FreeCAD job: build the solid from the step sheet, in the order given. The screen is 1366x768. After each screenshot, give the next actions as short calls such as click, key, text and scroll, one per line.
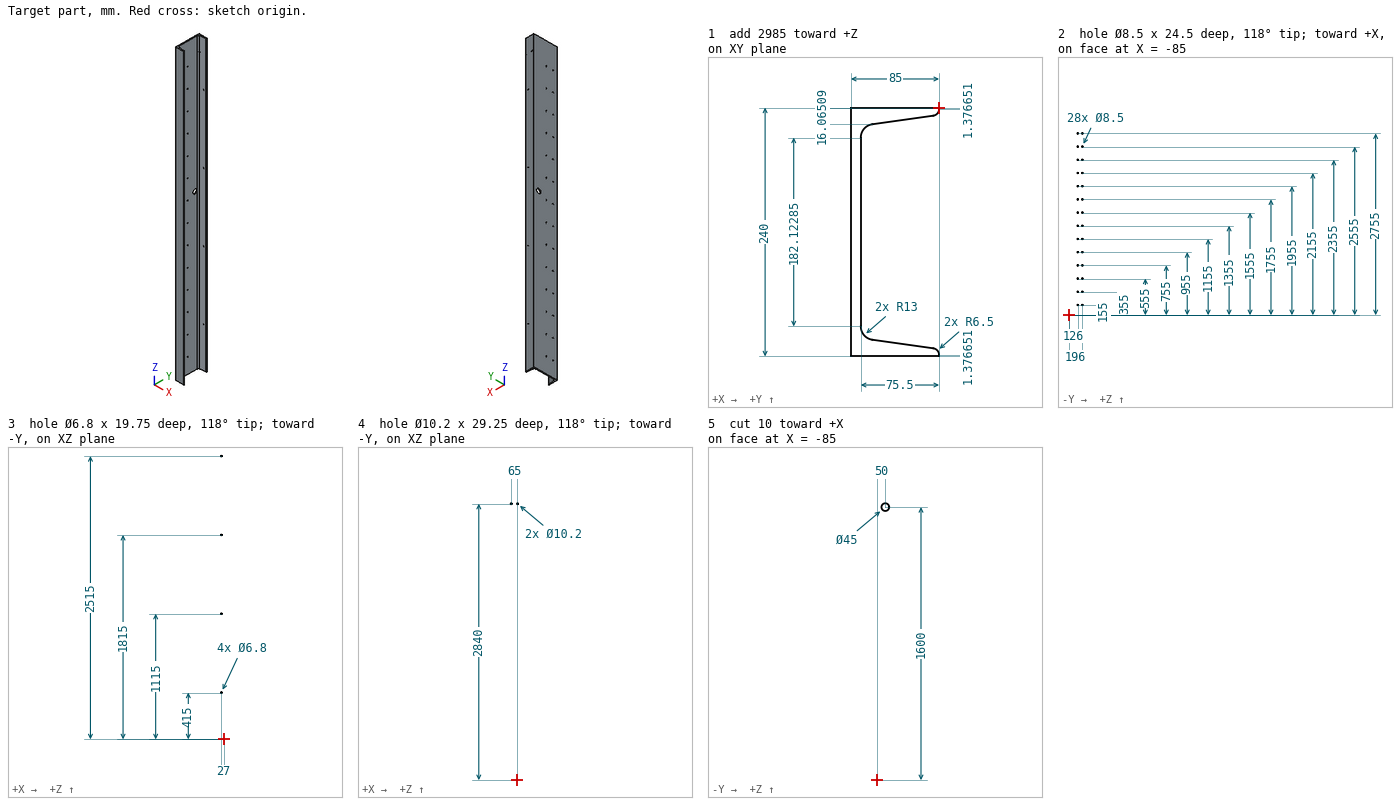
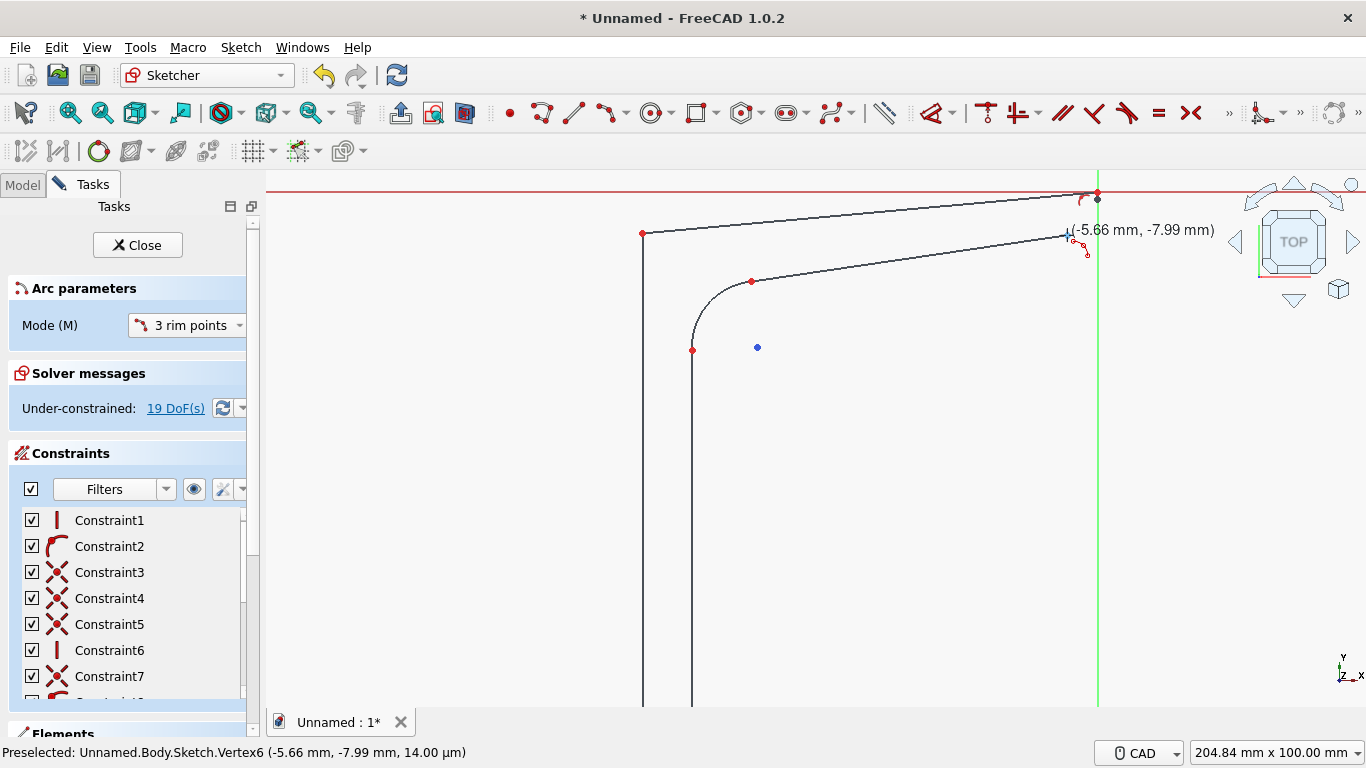
scroll(1098, 200, up, 8)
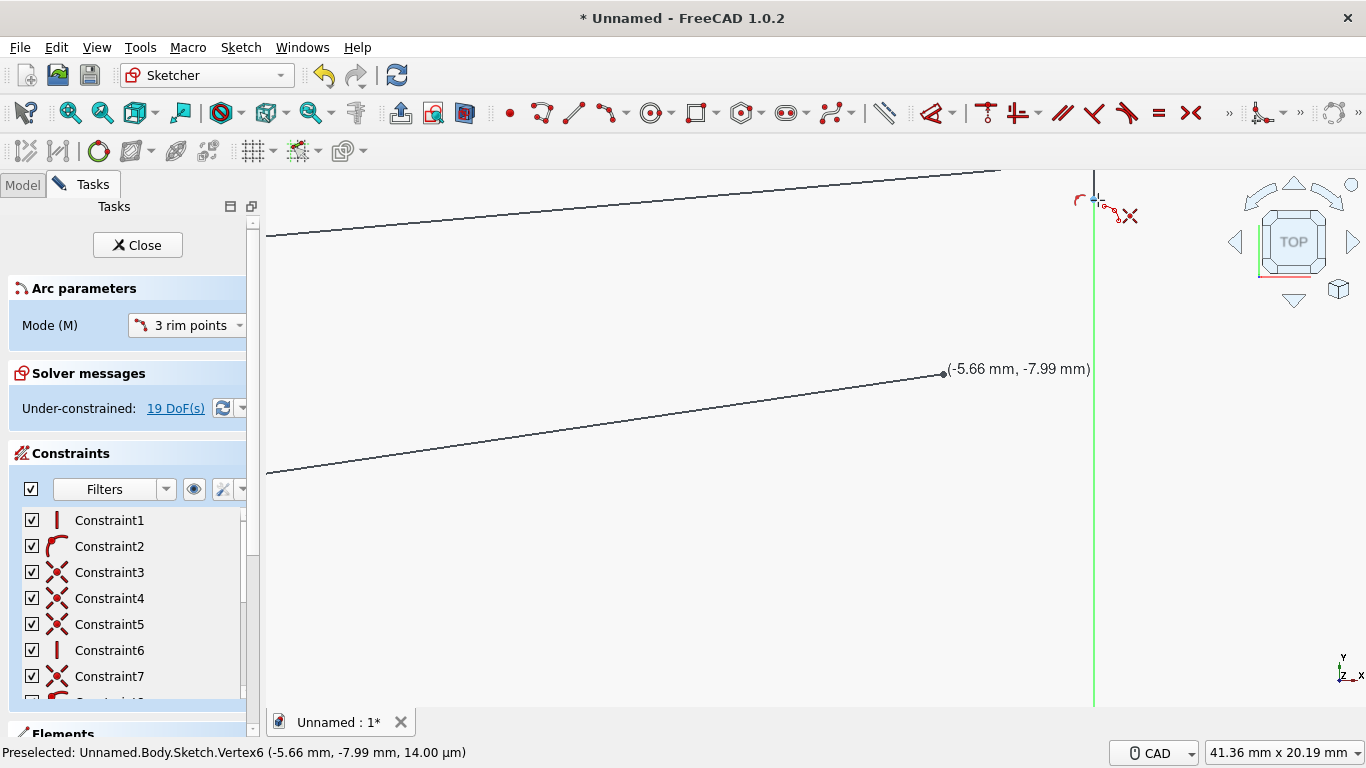
click(1094, 199)
click(1051, 312)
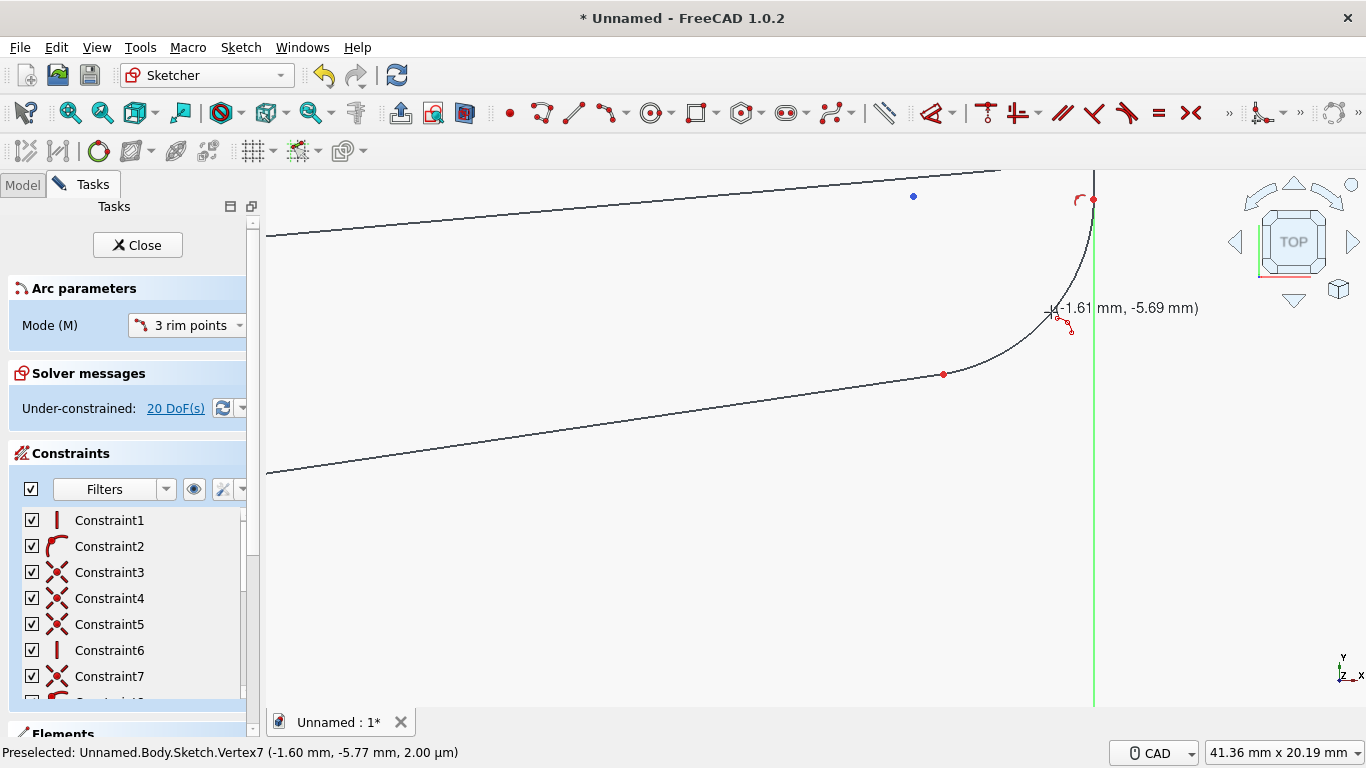
scroll(789, 286, down, 15)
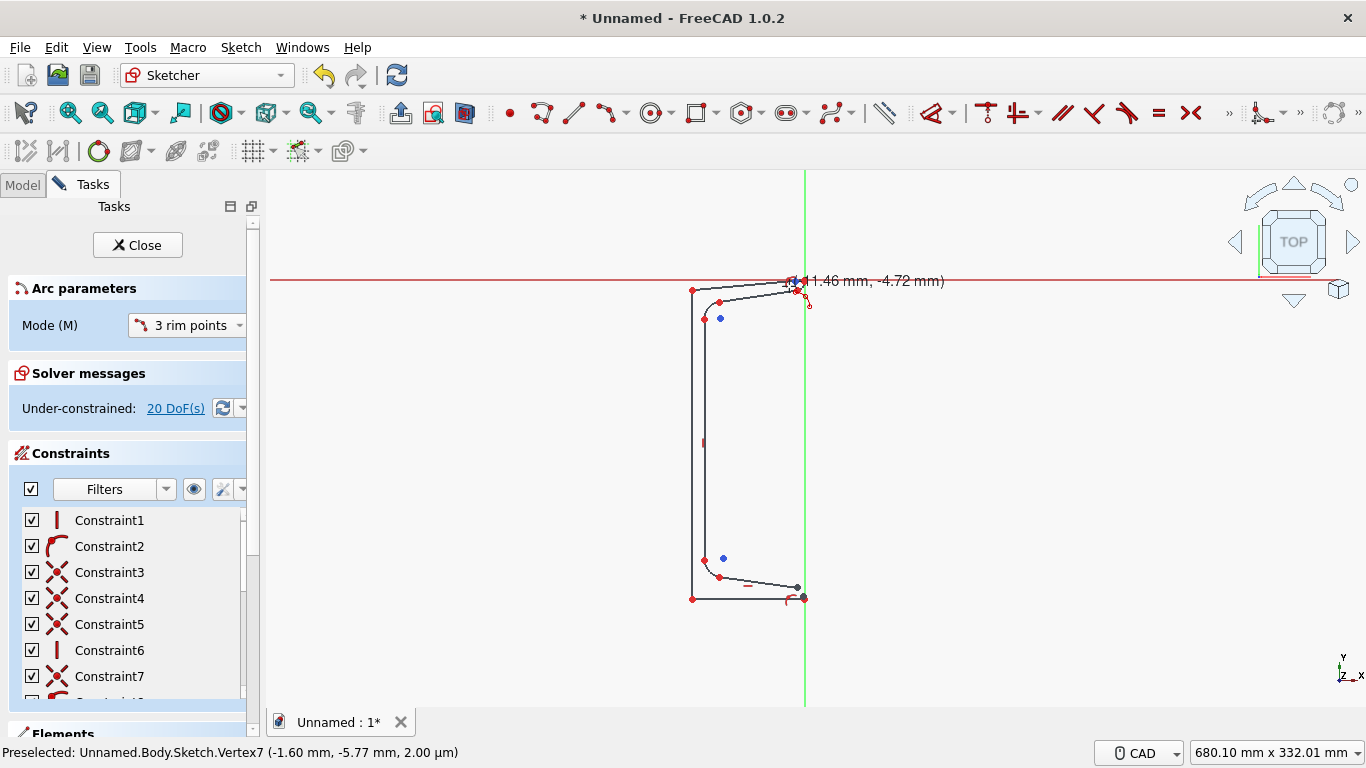
scroll(805, 596, up, 15)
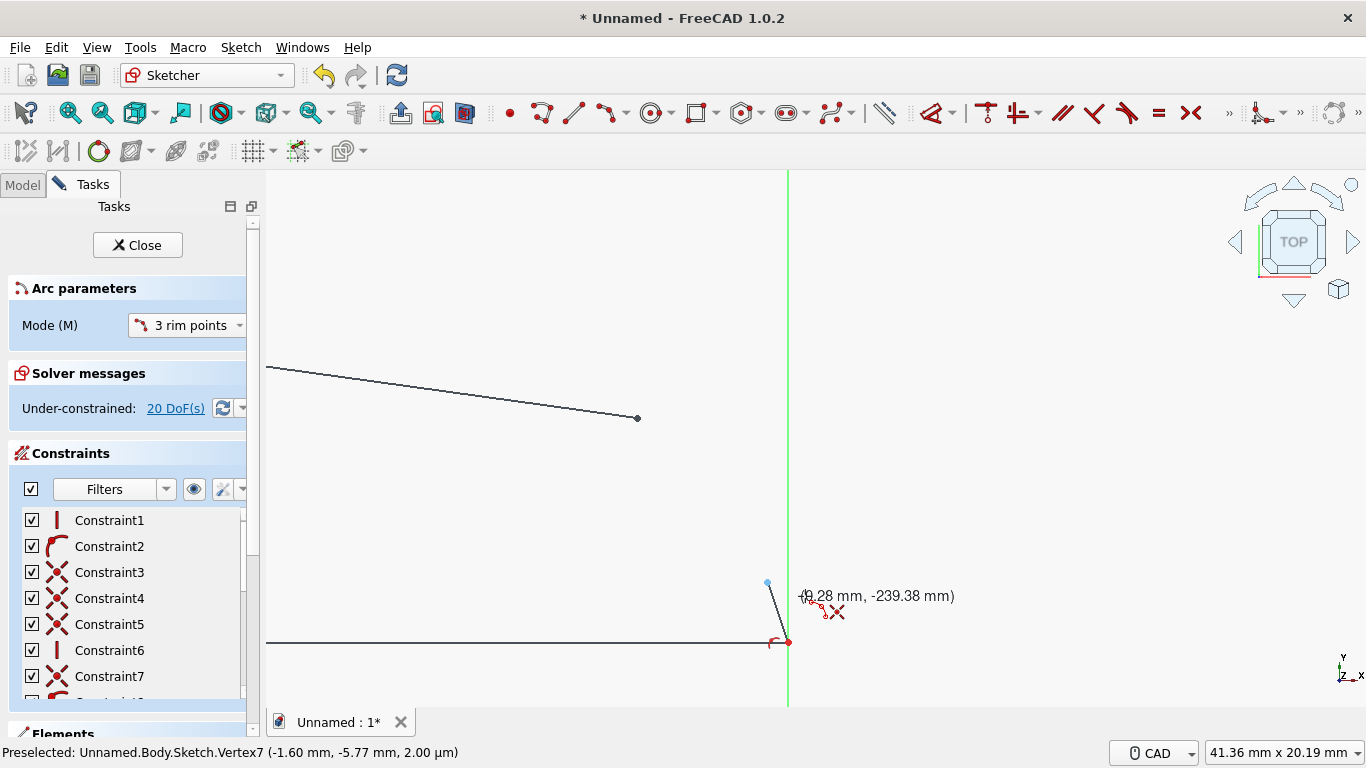
click(768, 582)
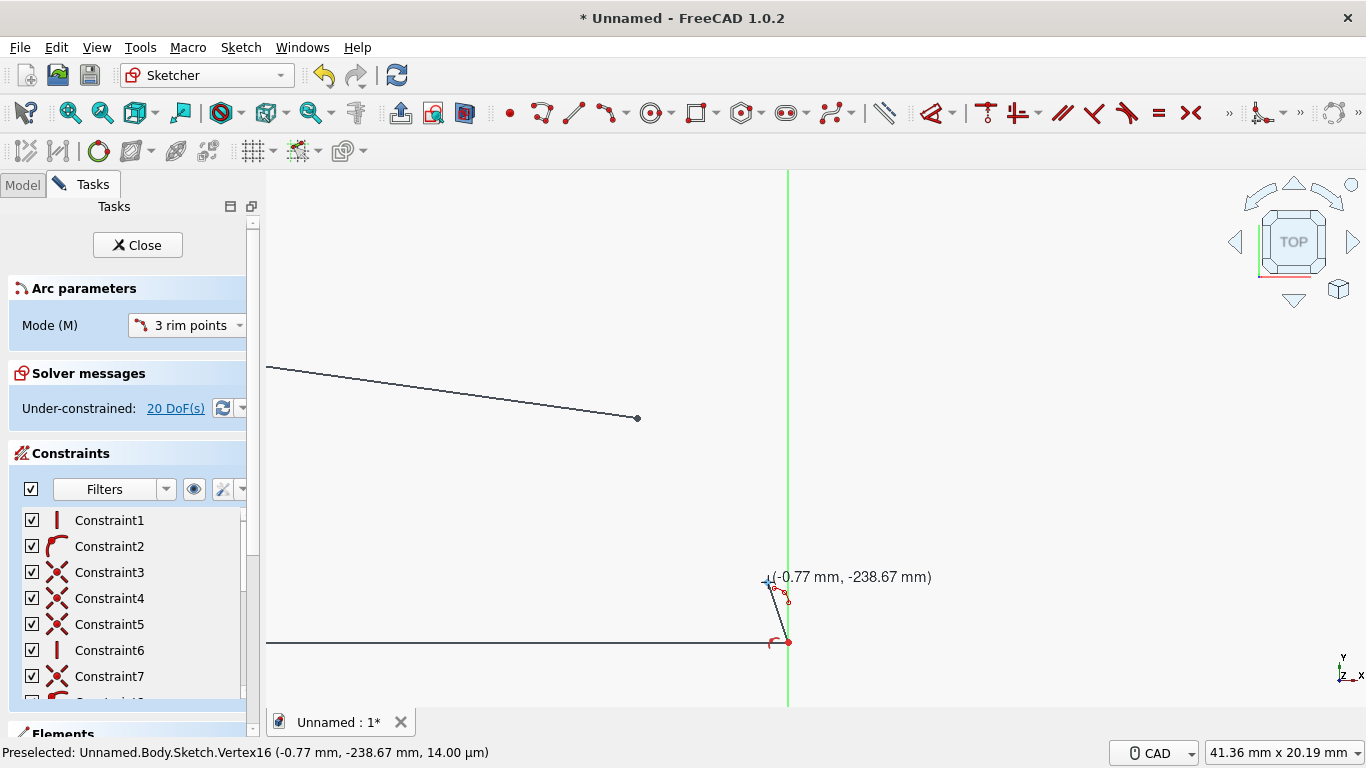
scroll(805, 596, down, 15)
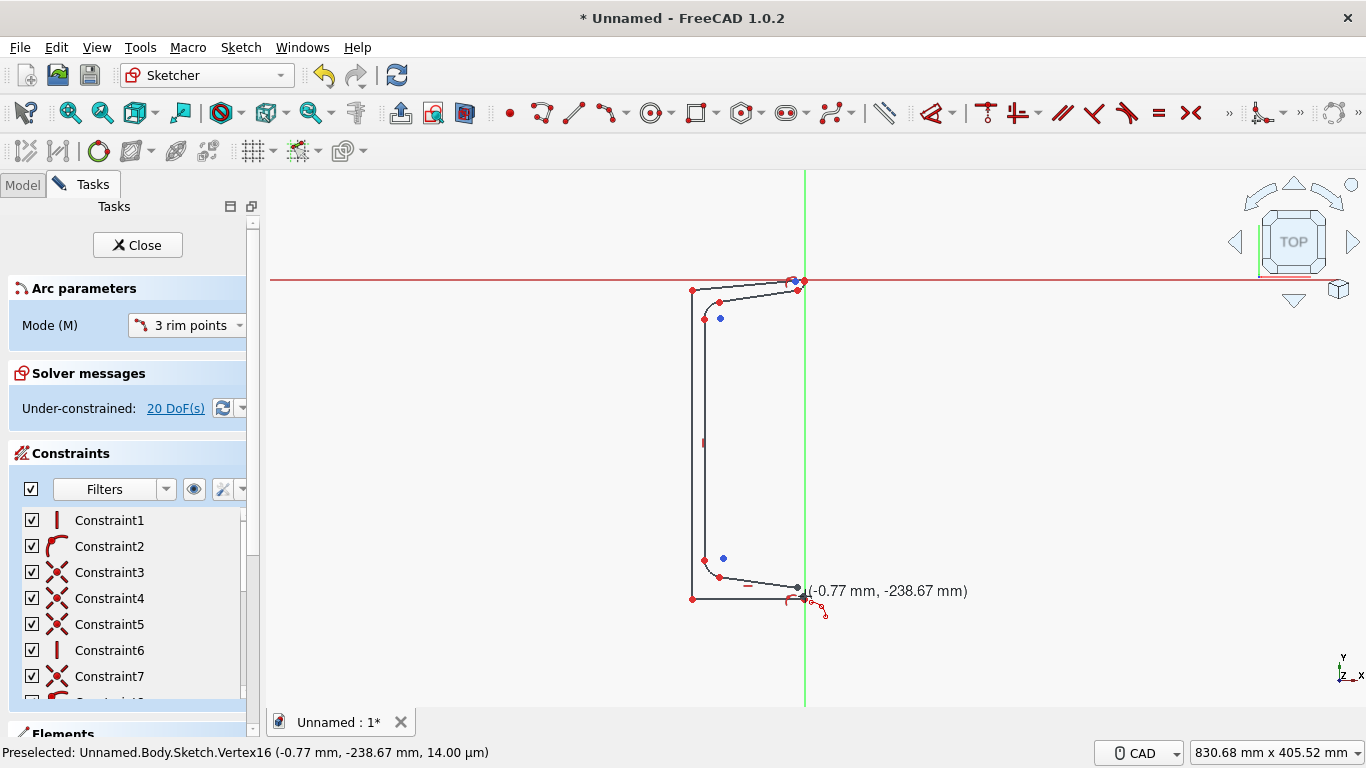
scroll(797, 587, up, 4)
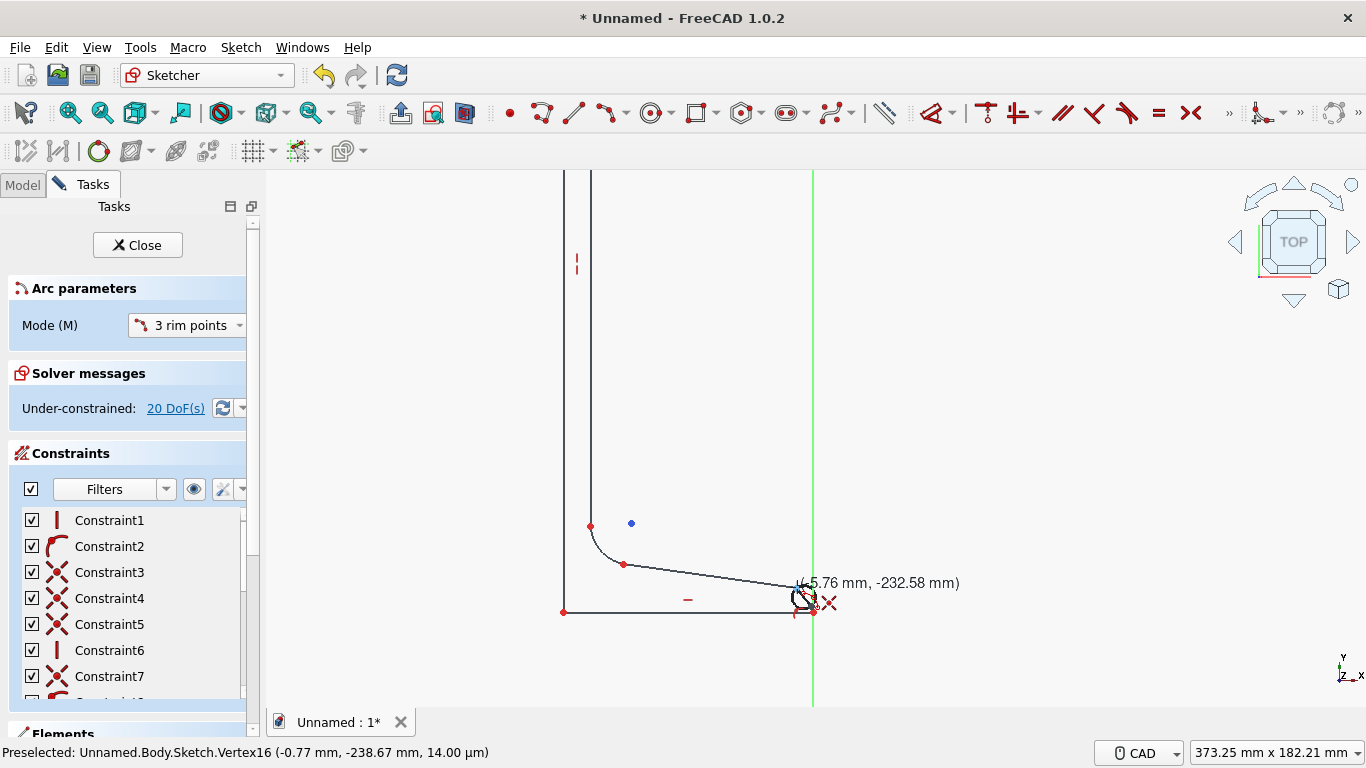
click(797, 588)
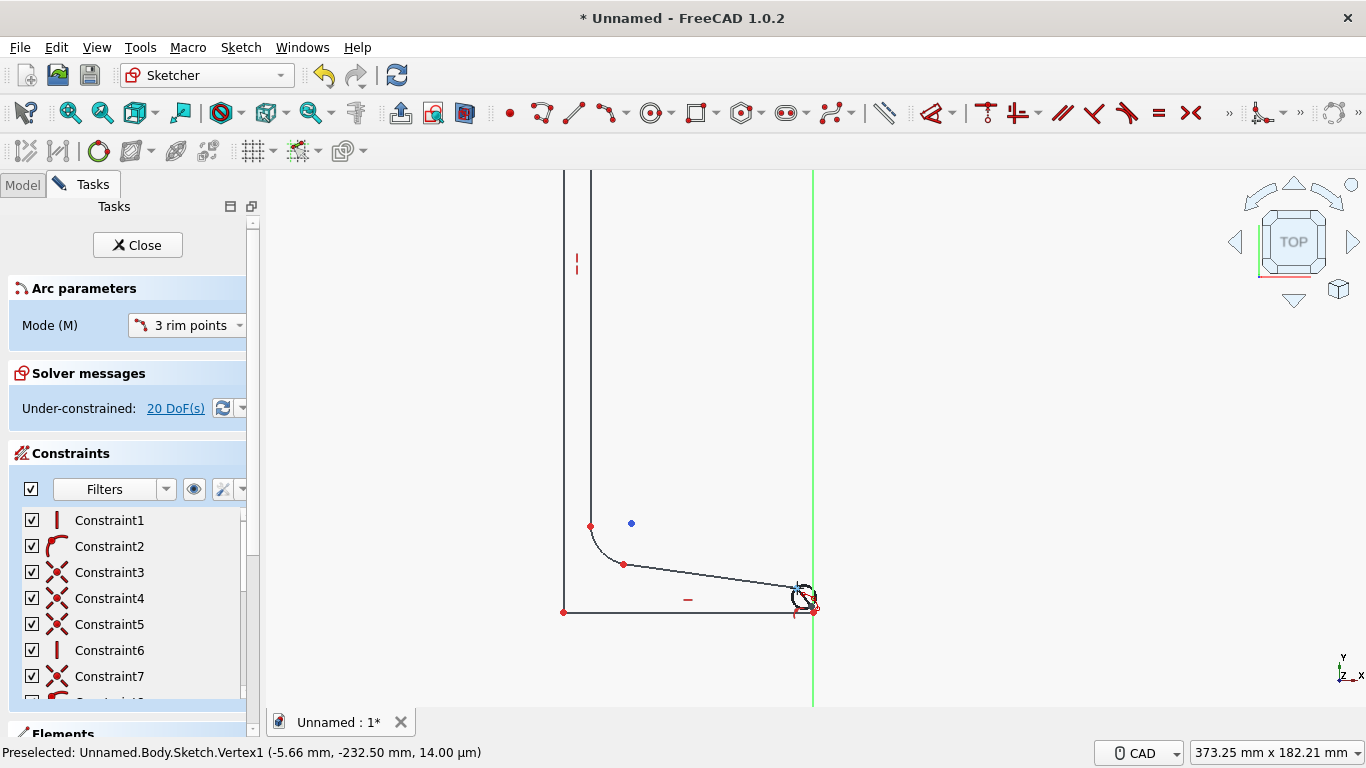
scroll(809, 594, up, 7)